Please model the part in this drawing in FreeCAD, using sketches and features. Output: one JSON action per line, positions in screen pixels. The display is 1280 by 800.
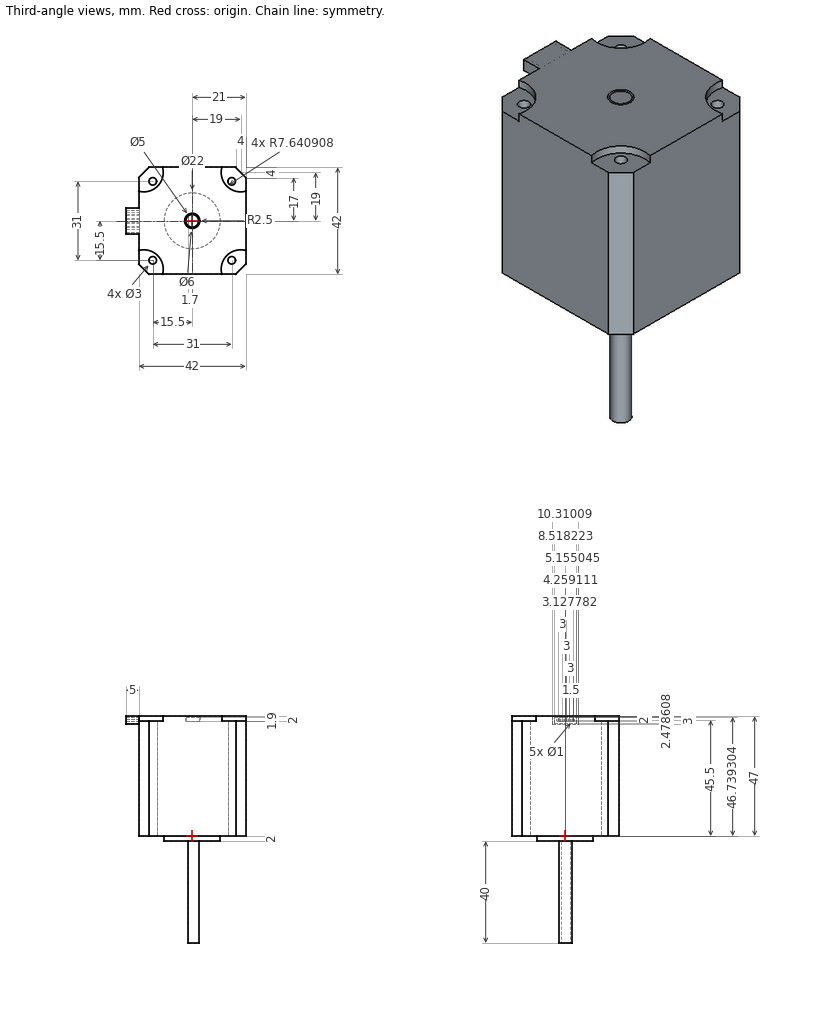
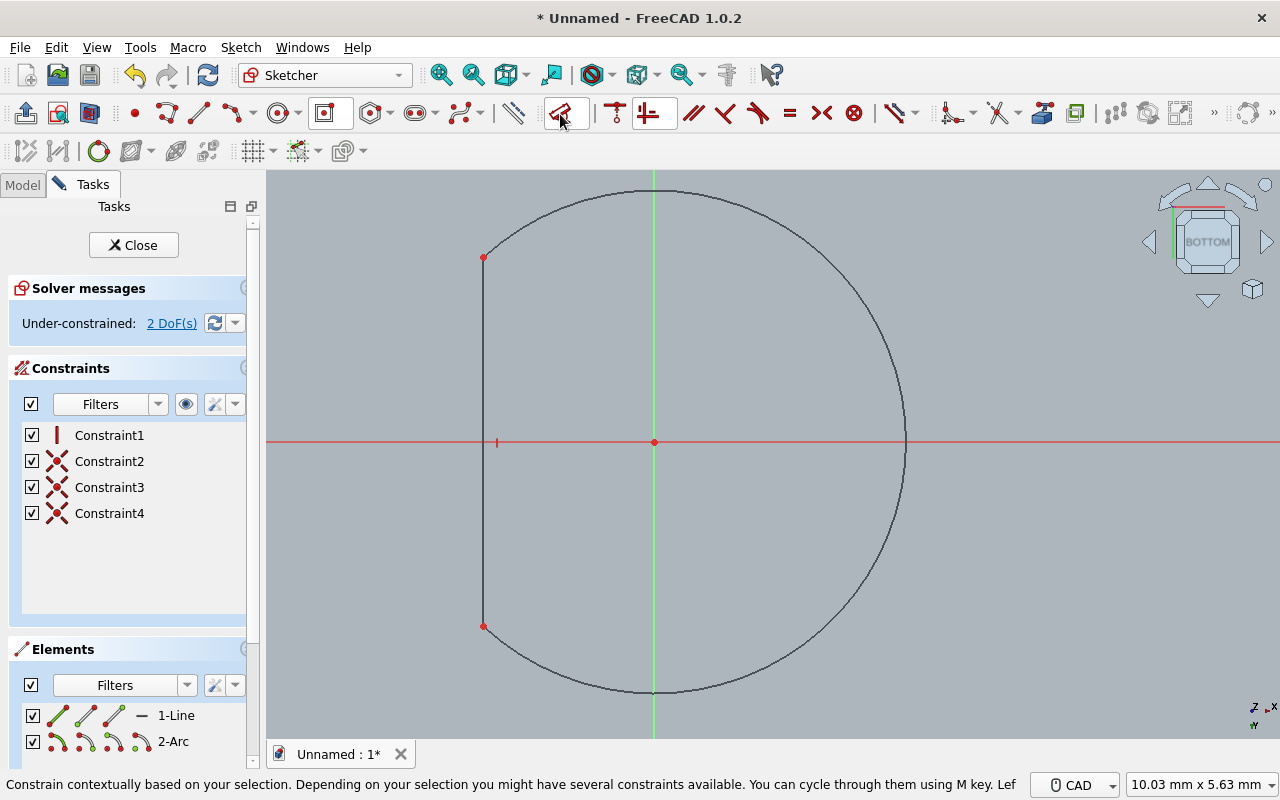
{"action": "left_click", "coordinate": [805, 643]}
{"action": "left_click", "coordinate": [824, 669]}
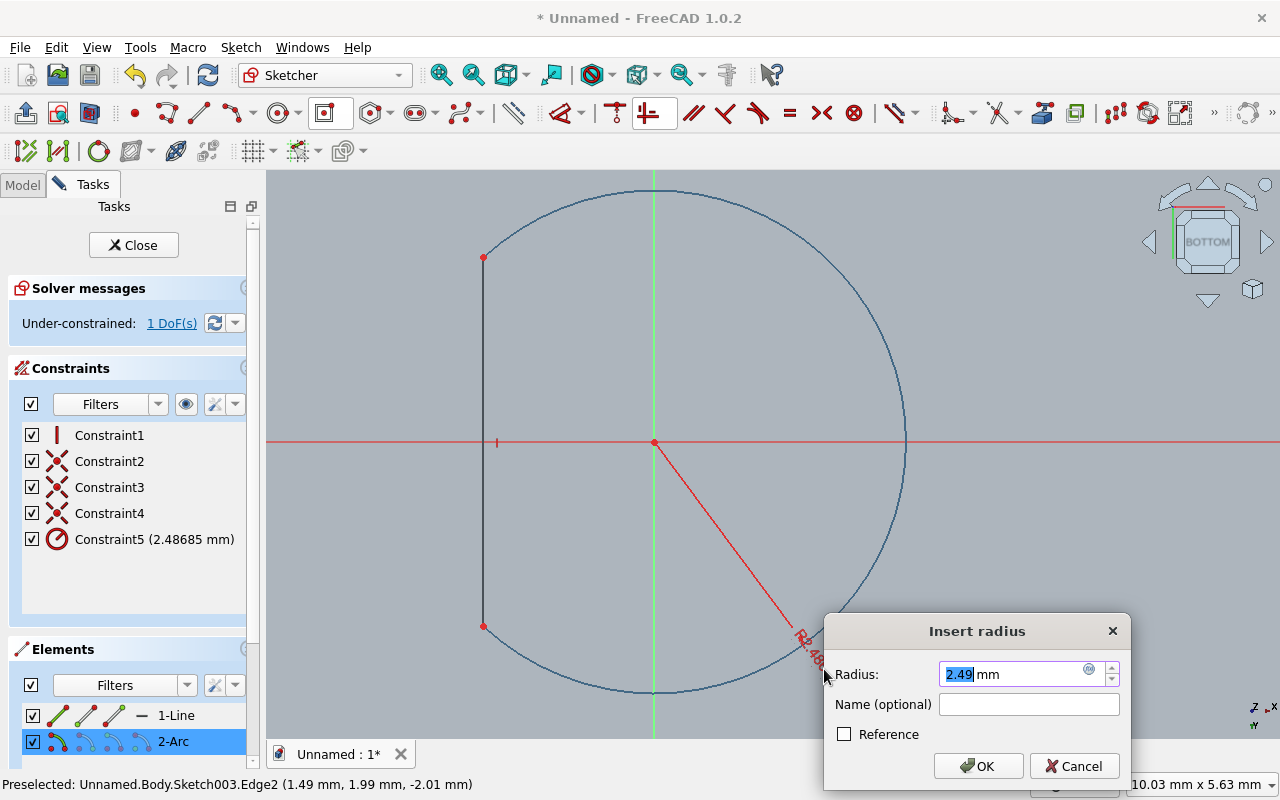
{"action": "type", "text": "2.5"}
{"action": "key", "text": "Return"}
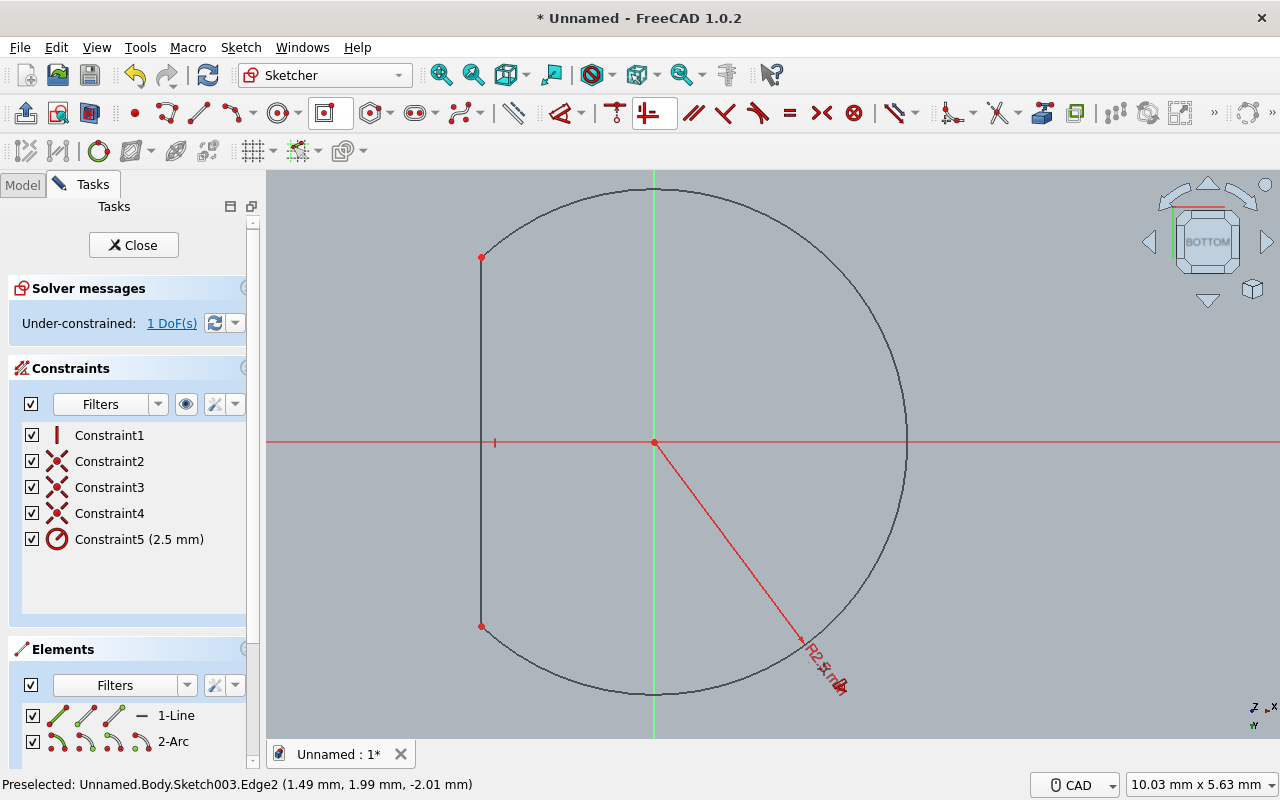
{"action": "left_click", "coordinate": [481, 258]}
{"action": "left_click", "coordinate": [568, 224]}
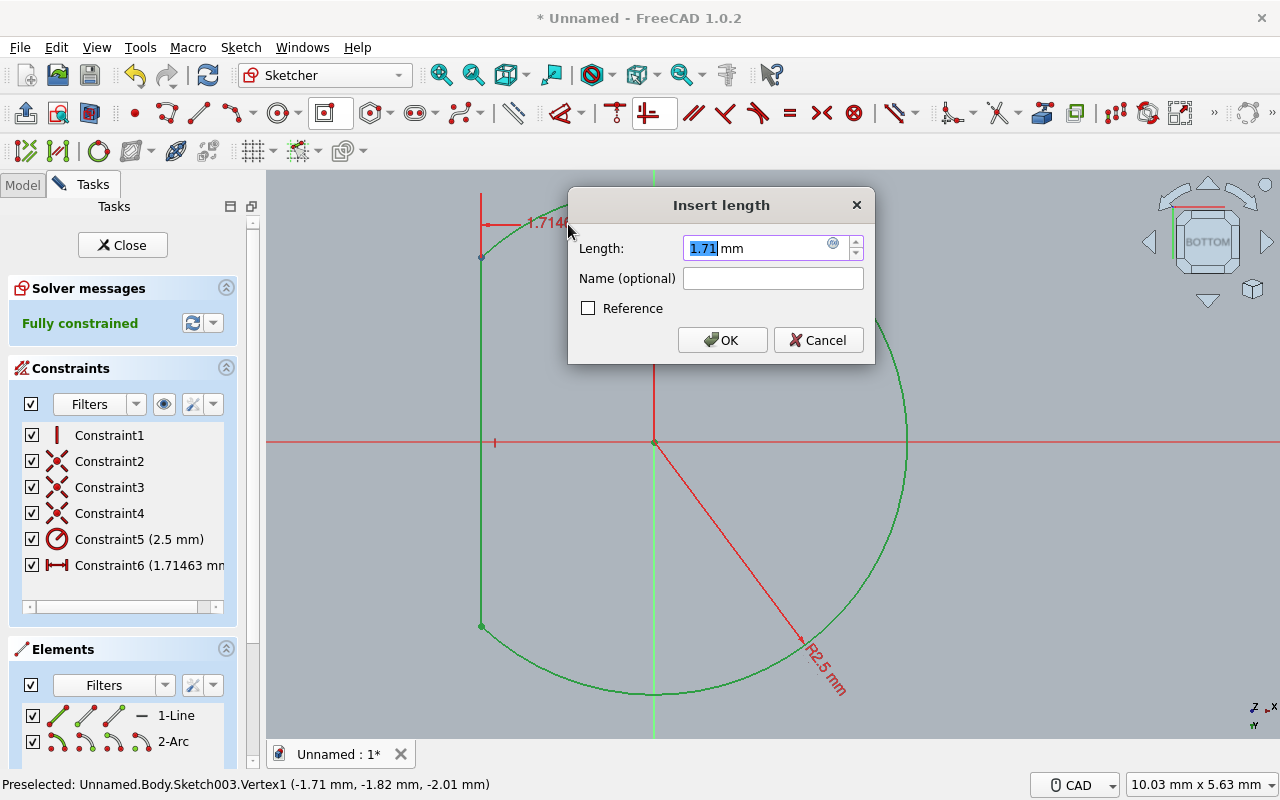
{"action": "type", "text": "1.7"}
{"action": "key", "text": "Return"}
{"action": "key", "text": "Escape"}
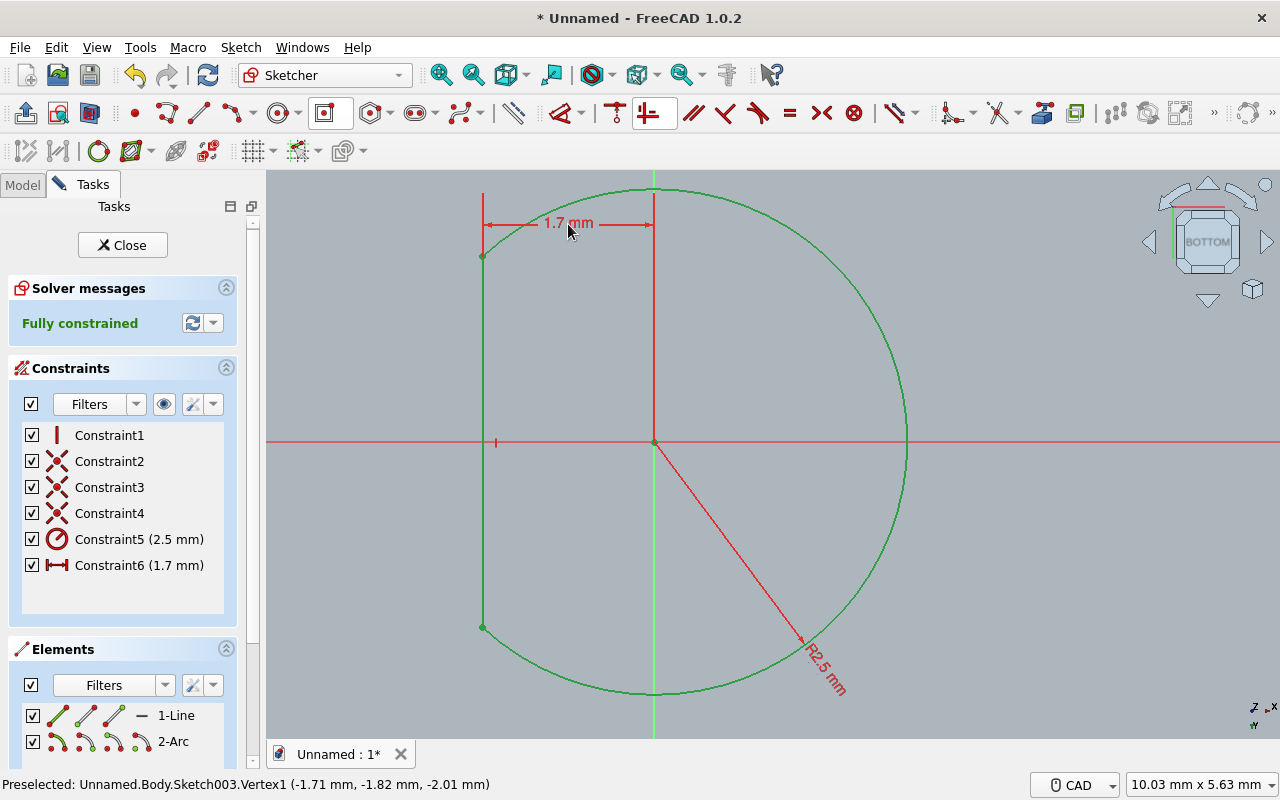
{"action": "left_click", "coordinate": [123, 245]}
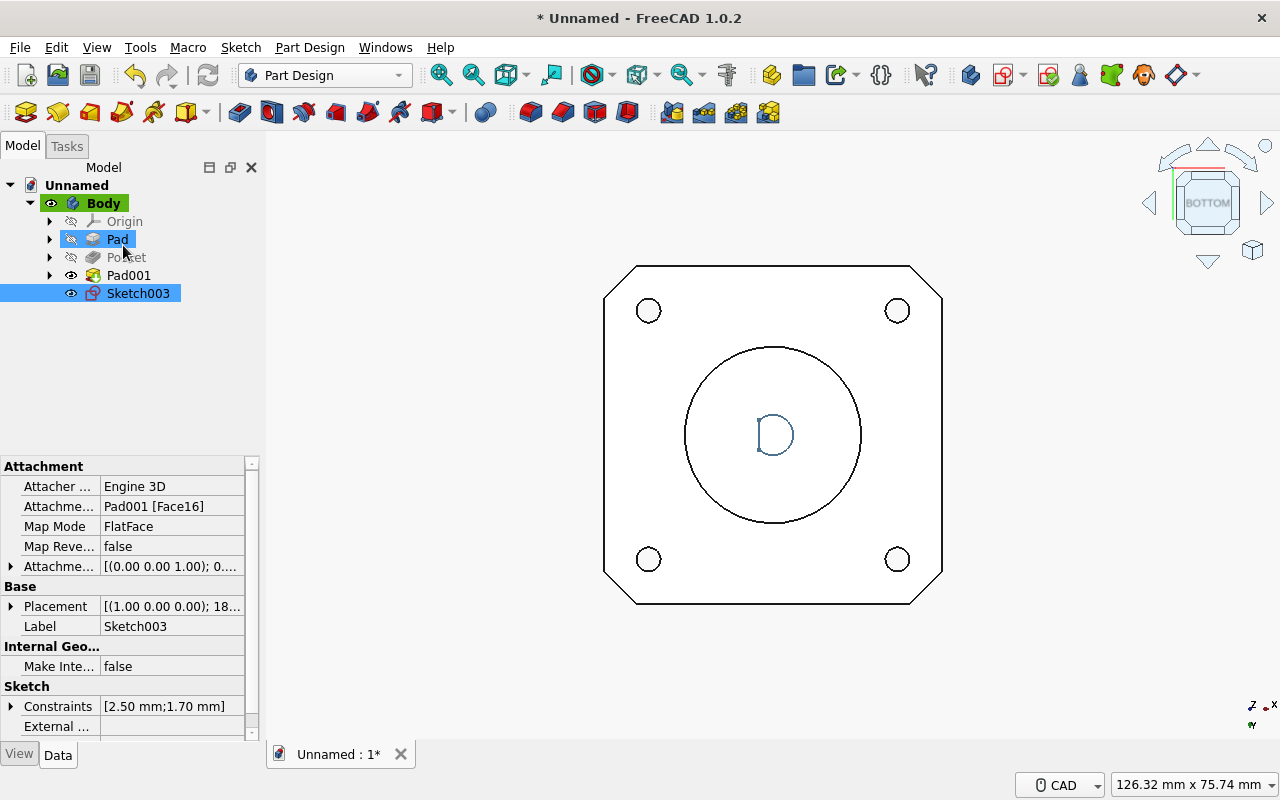
{"action": "left_click", "coordinate": [26, 112]}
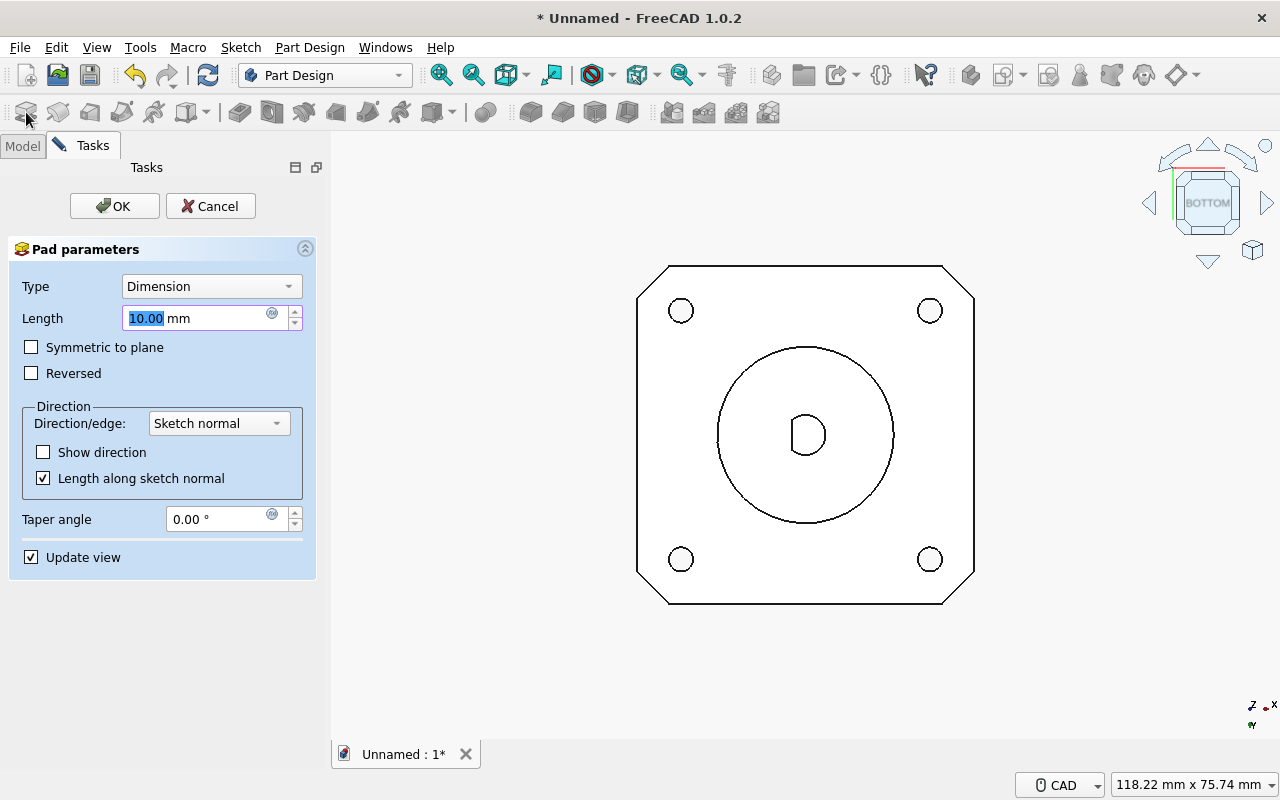
{"action": "type", "text": "40"}
{"action": "key", "text": "Tab"}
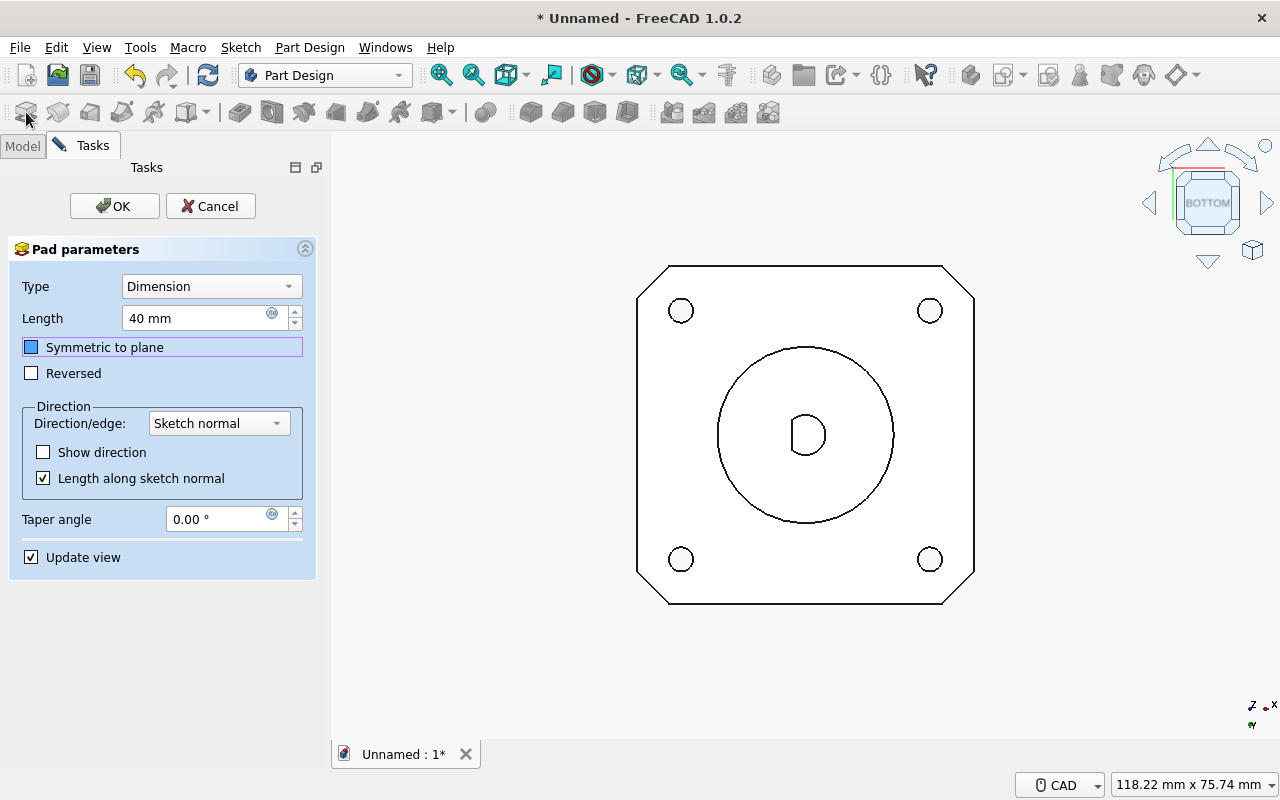
{"action": "left_click", "coordinate": [115, 206]}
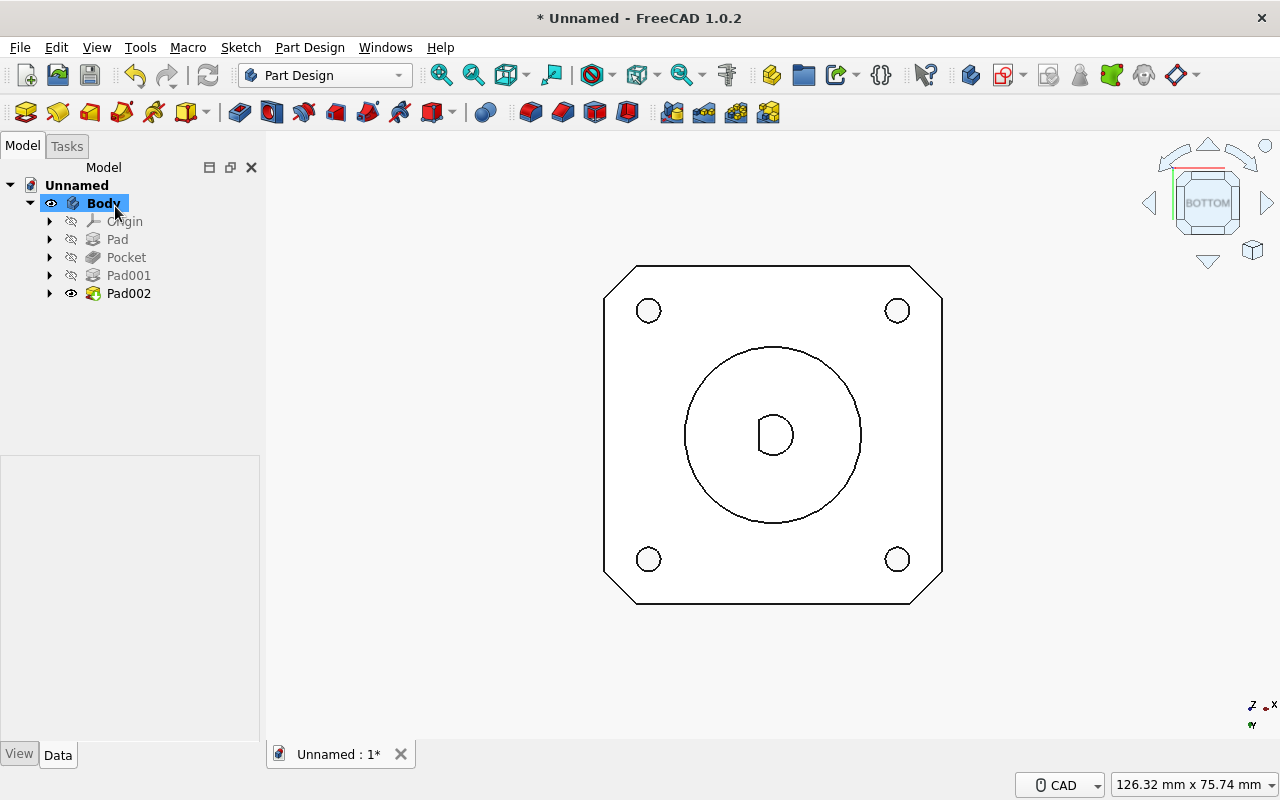
{"action": "key", "text": "0"}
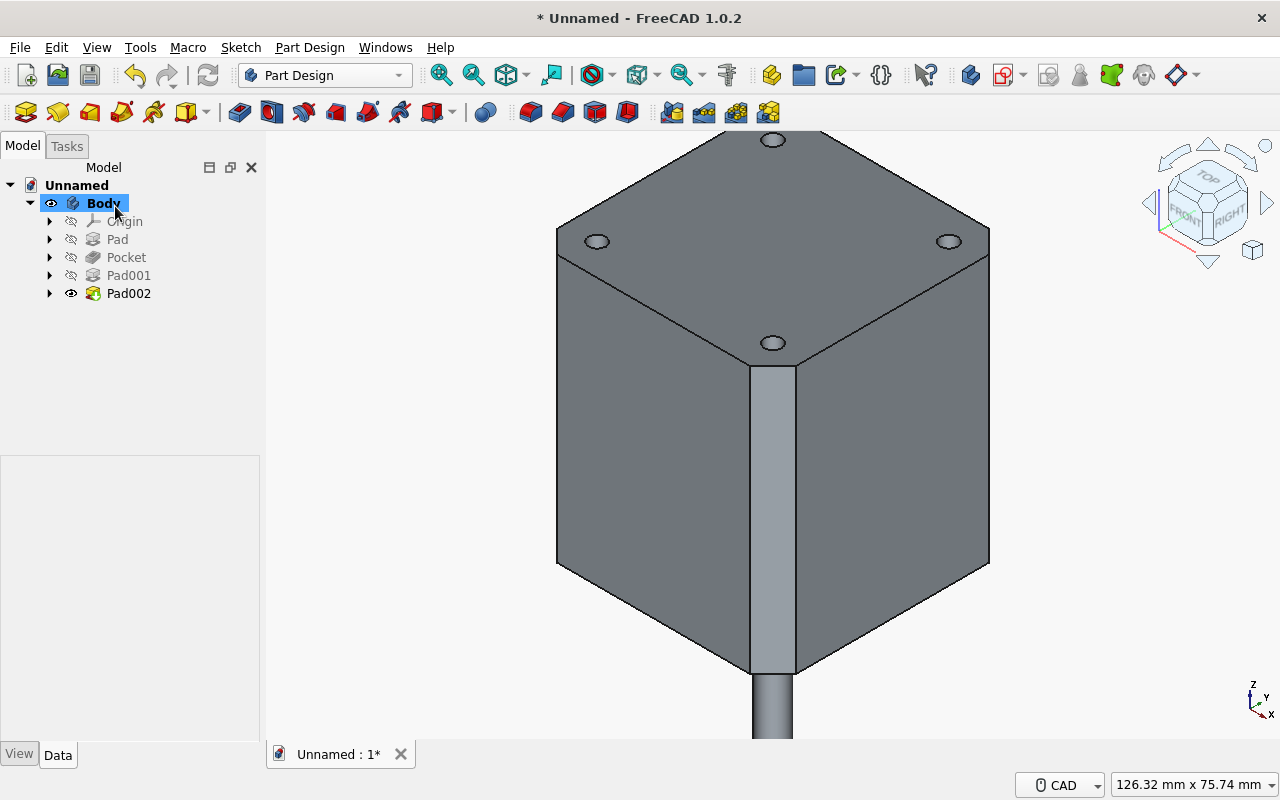
{"action": "key", "text": "v f"}